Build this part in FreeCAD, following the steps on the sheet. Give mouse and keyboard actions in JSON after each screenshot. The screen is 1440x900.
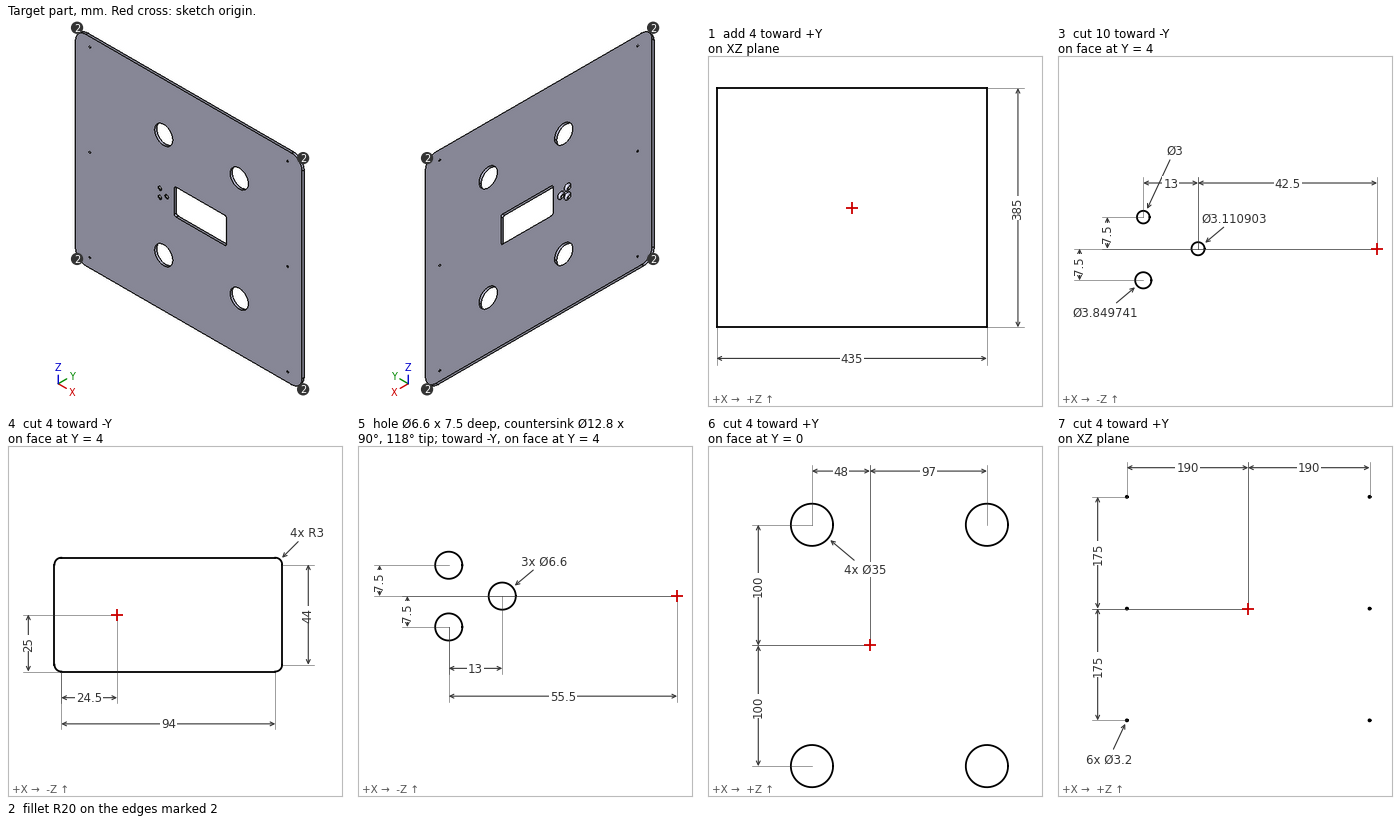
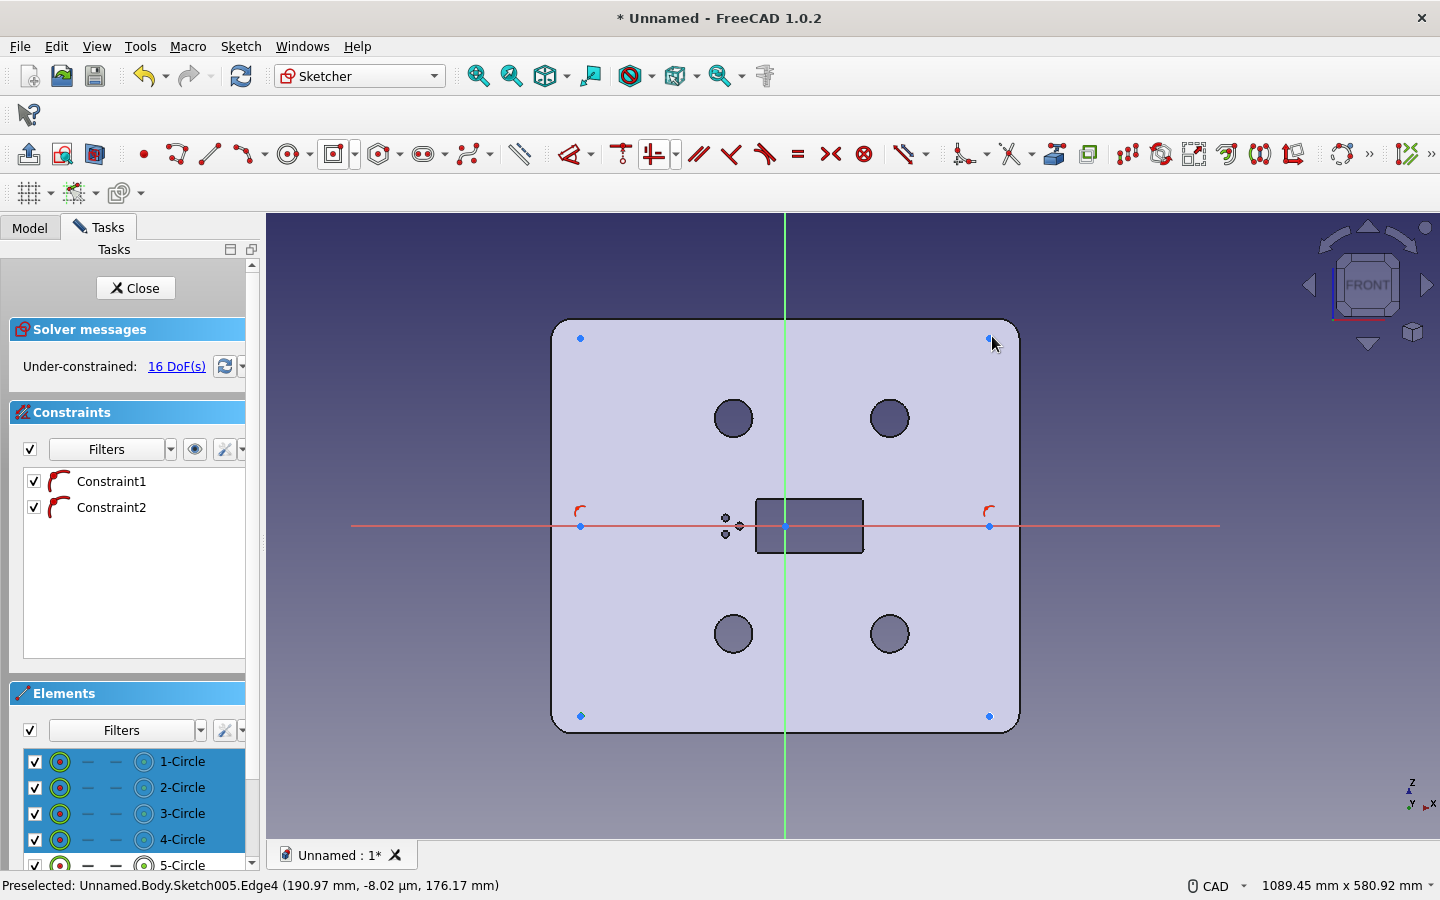
{"action": "scroll", "coordinate": [991, 525], "scroll_direction": "up", "scroll_amount": 12}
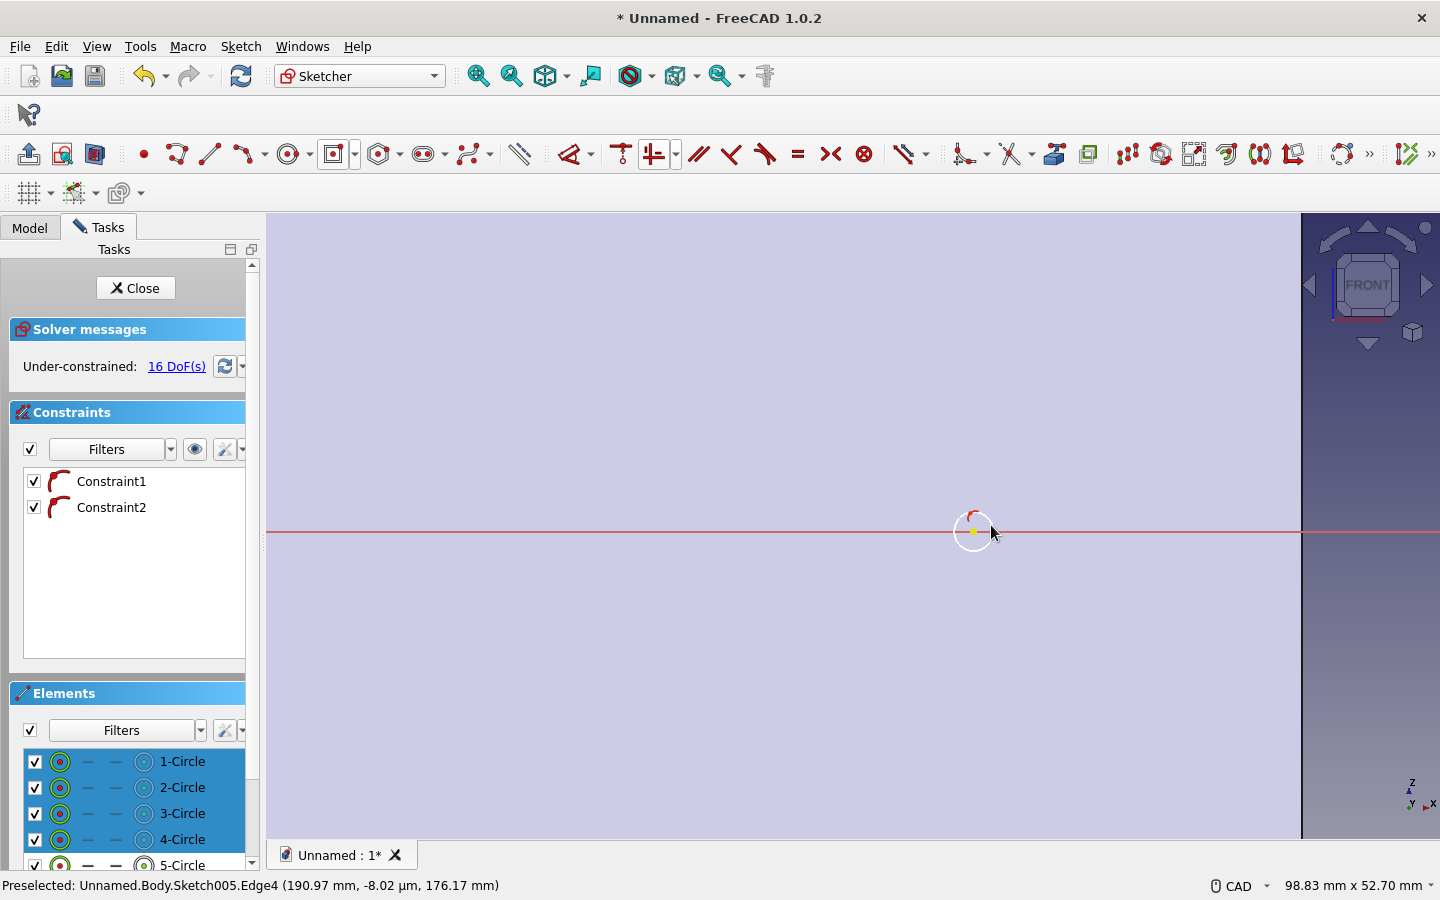
{"action": "left_click", "coordinate": [988, 518]}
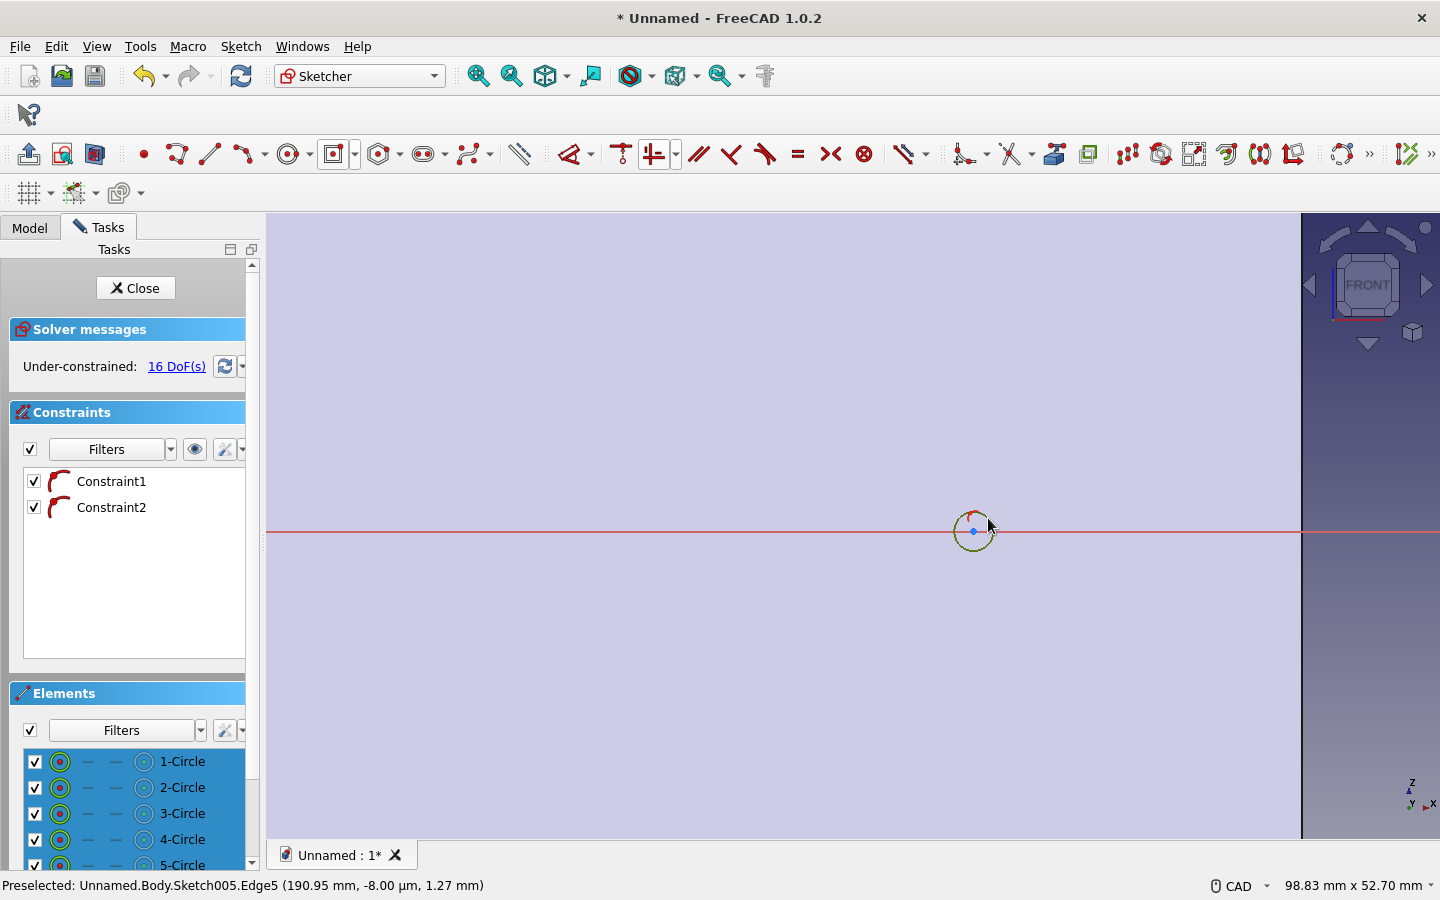
{"action": "scroll", "coordinate": [991, 525], "scroll_direction": "down", "scroll_amount": 12}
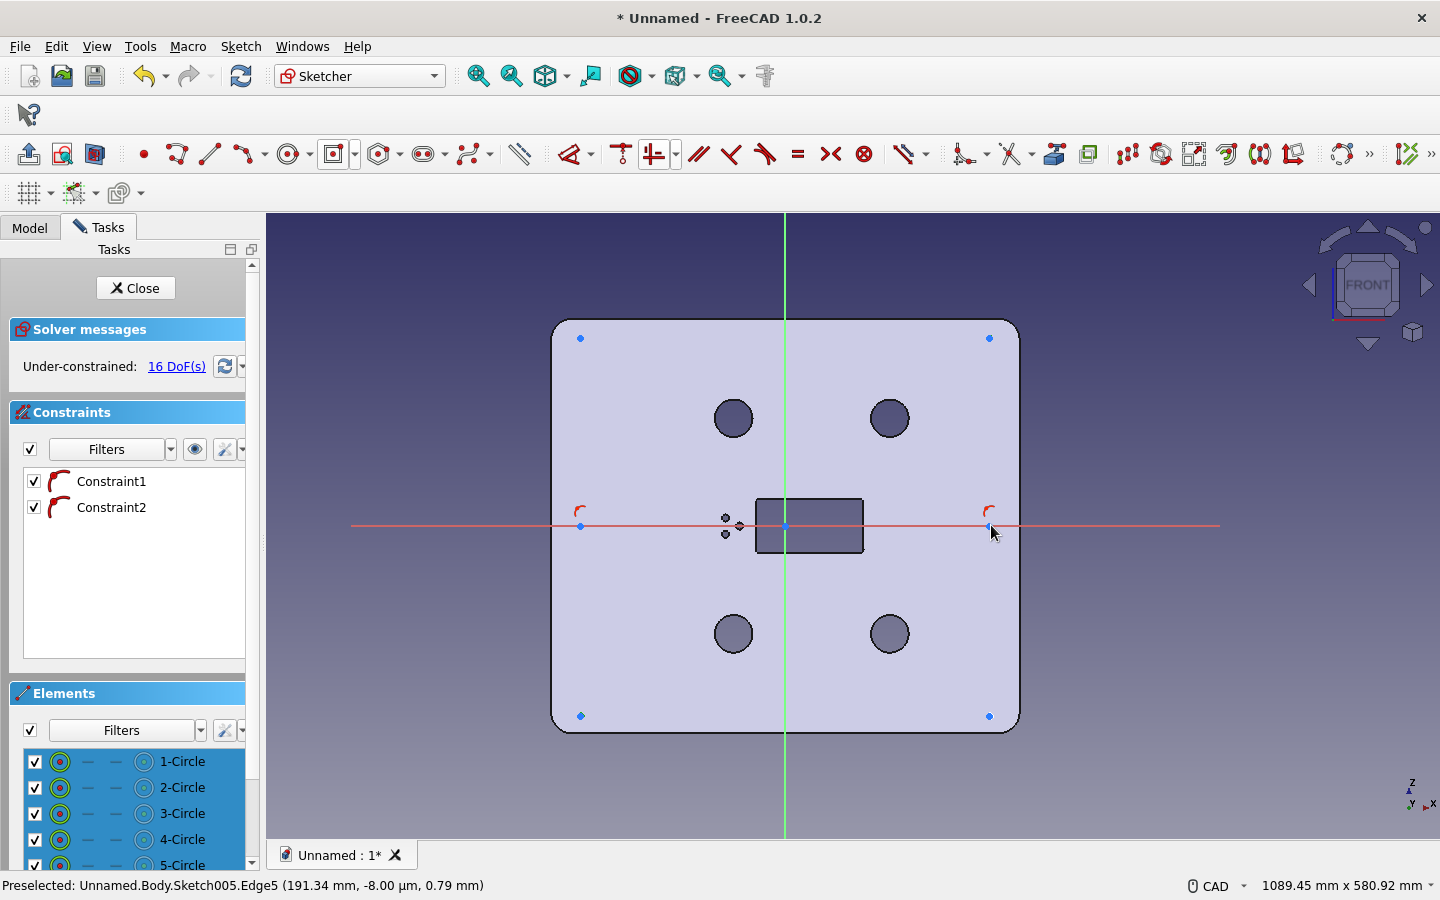
{"action": "scroll", "coordinate": [992, 714], "scroll_direction": "up", "scroll_amount": 8}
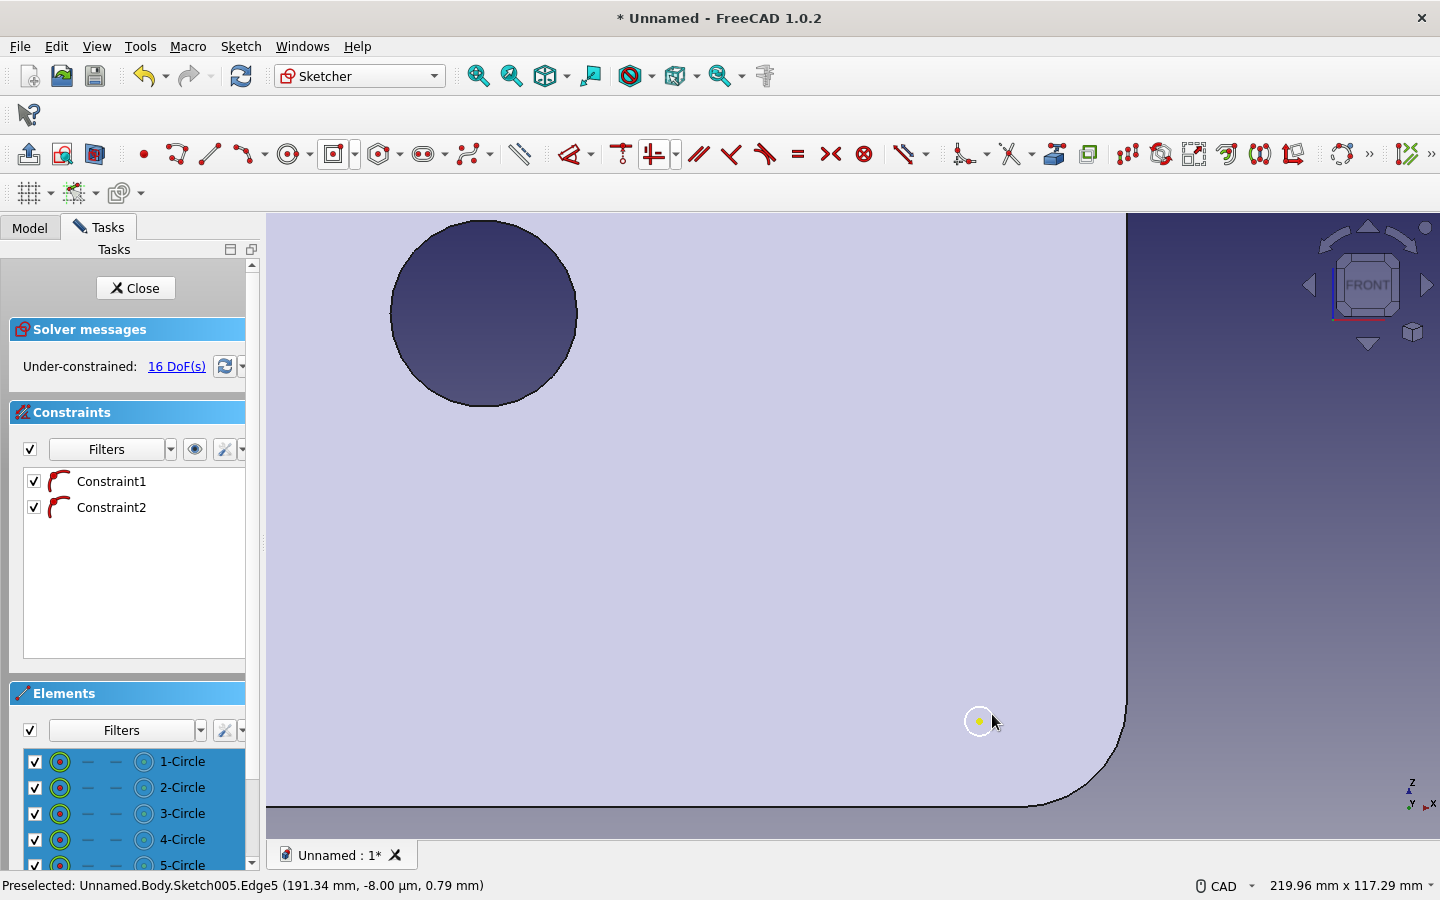
{"action": "left_click", "coordinate": [990, 711]}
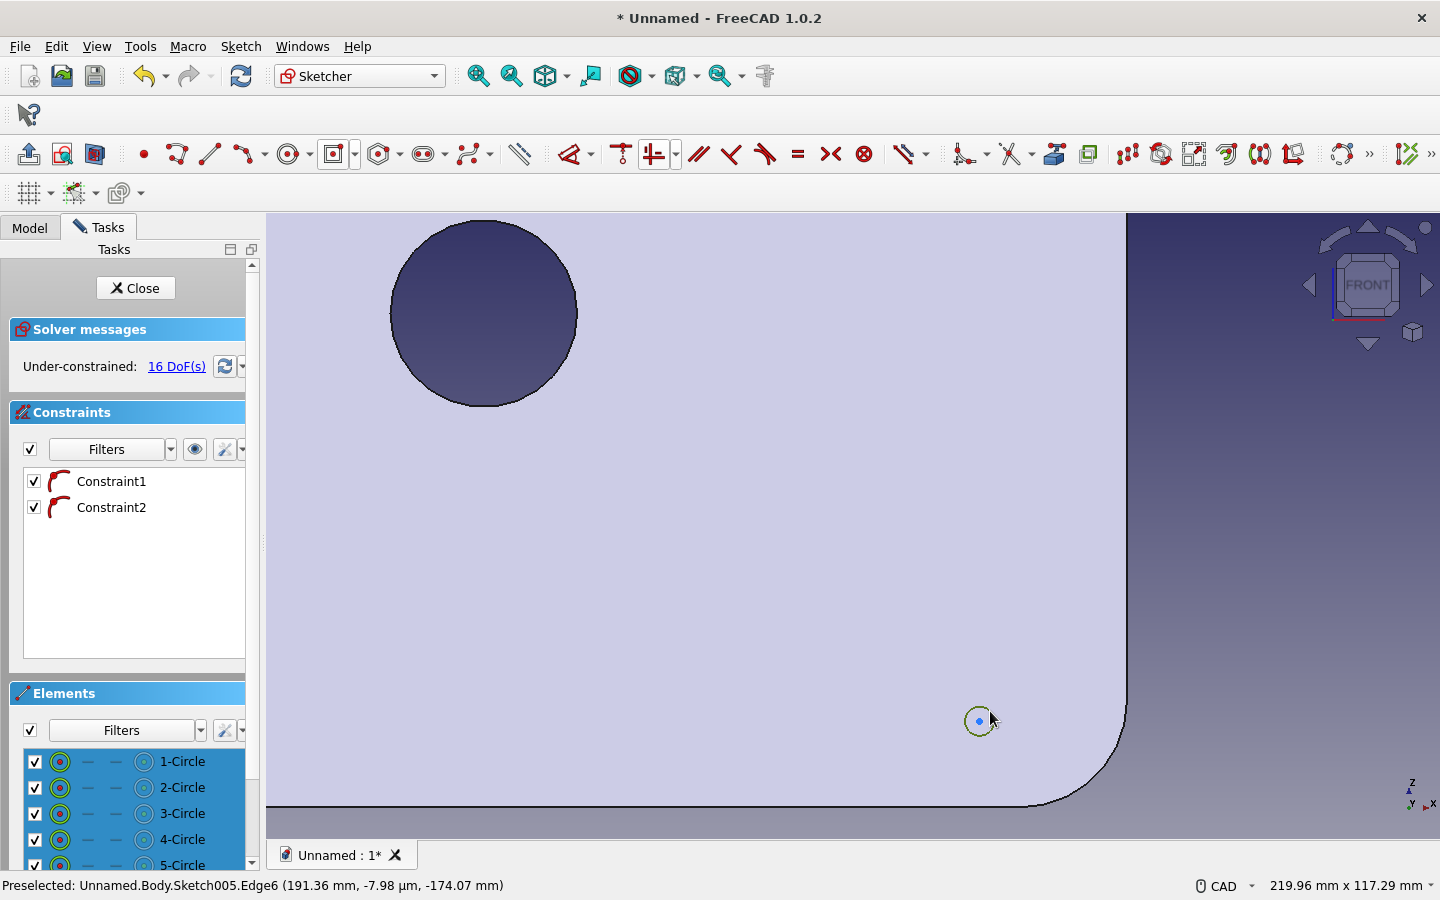
{"action": "left_click", "coordinate": [798, 154]}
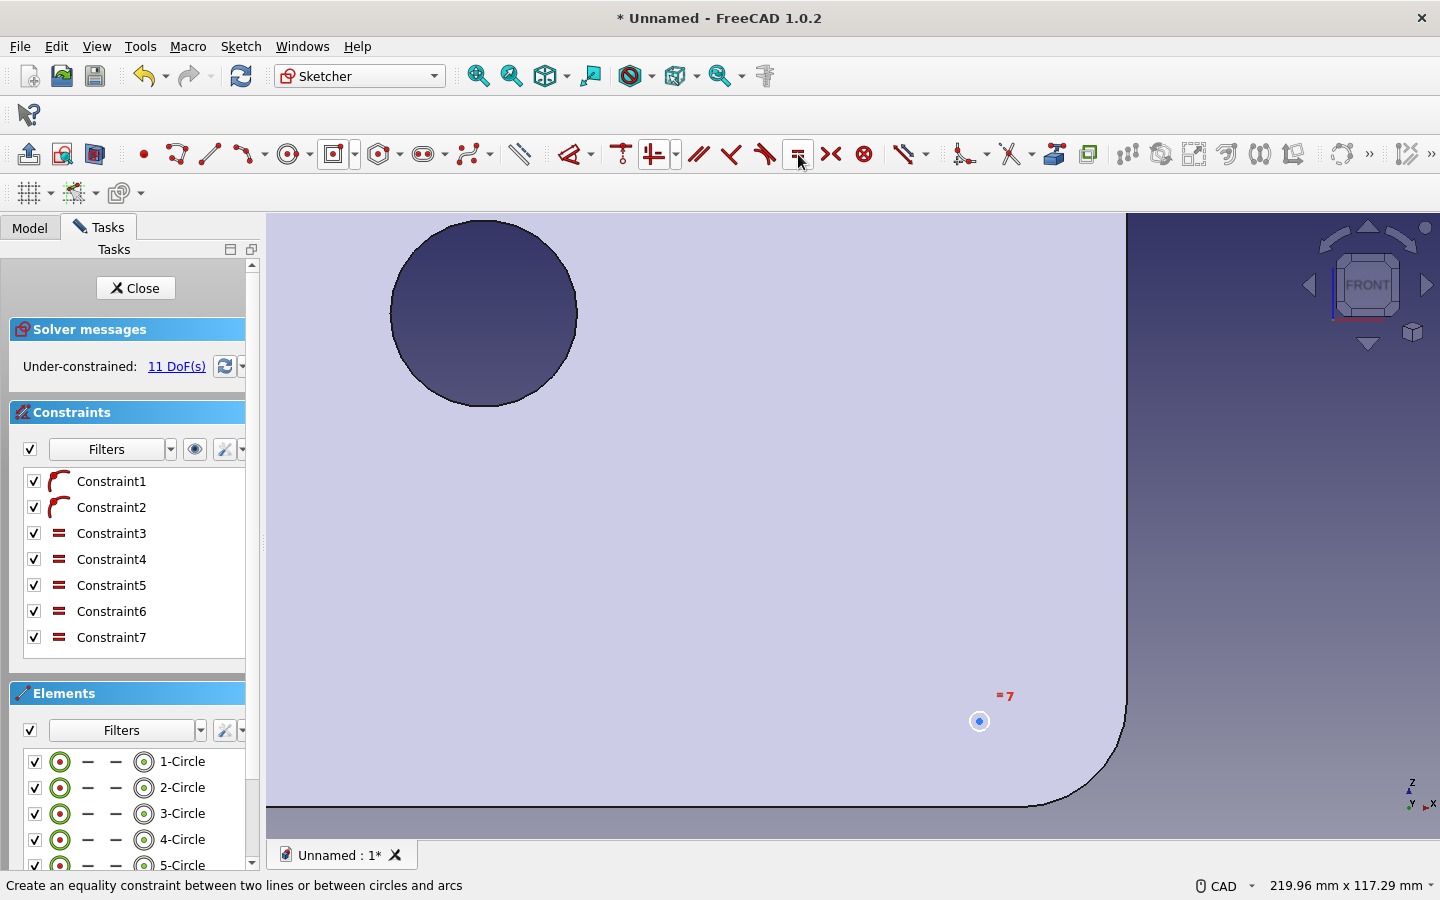
{"action": "scroll", "coordinate": [992, 715], "scroll_direction": "down", "scroll_amount": 8}